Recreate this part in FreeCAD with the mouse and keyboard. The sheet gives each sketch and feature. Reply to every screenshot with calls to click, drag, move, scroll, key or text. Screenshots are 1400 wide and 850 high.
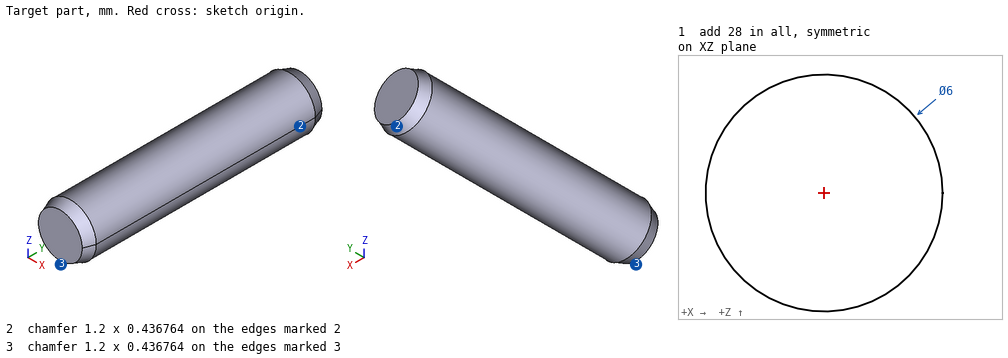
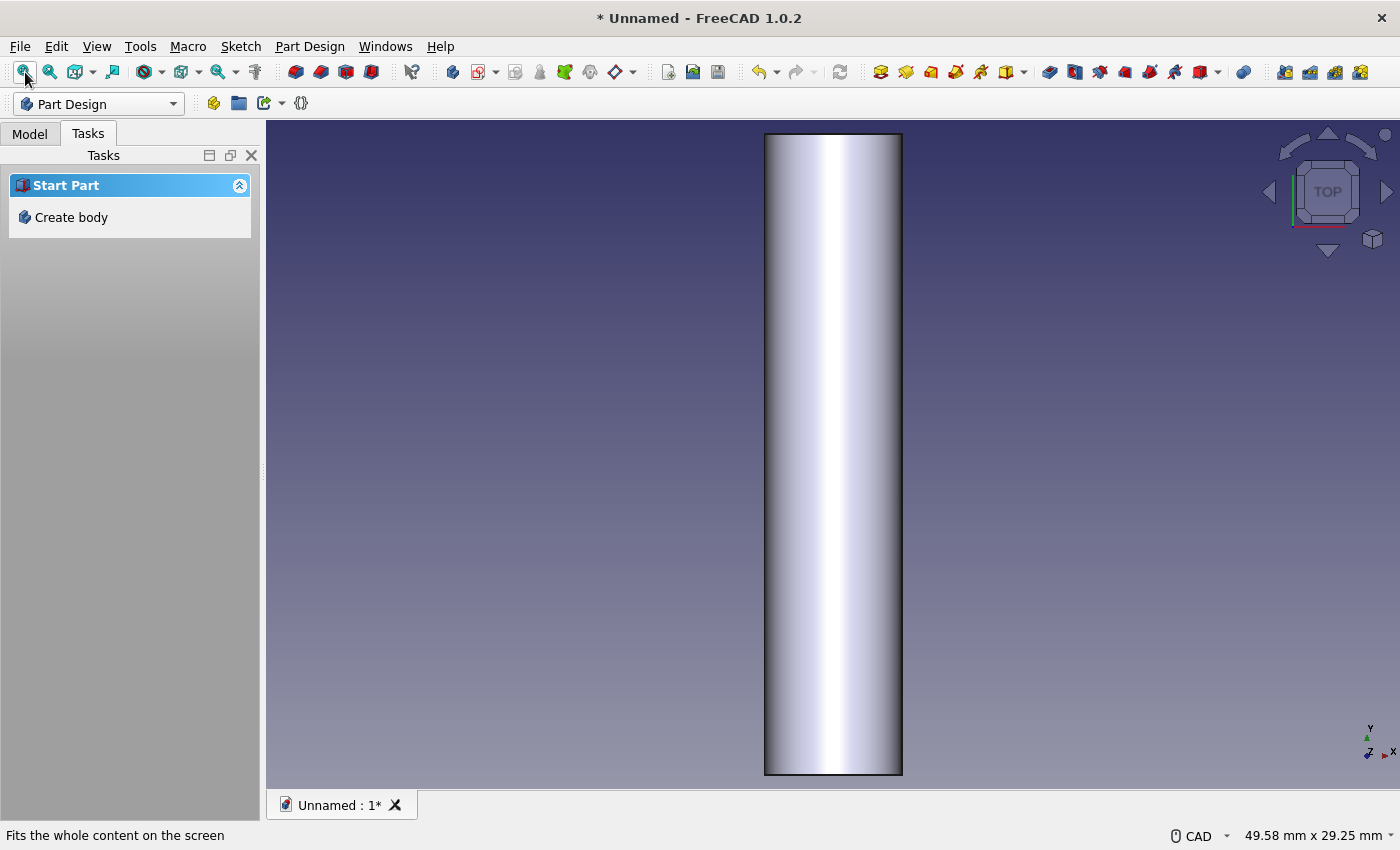
key(1)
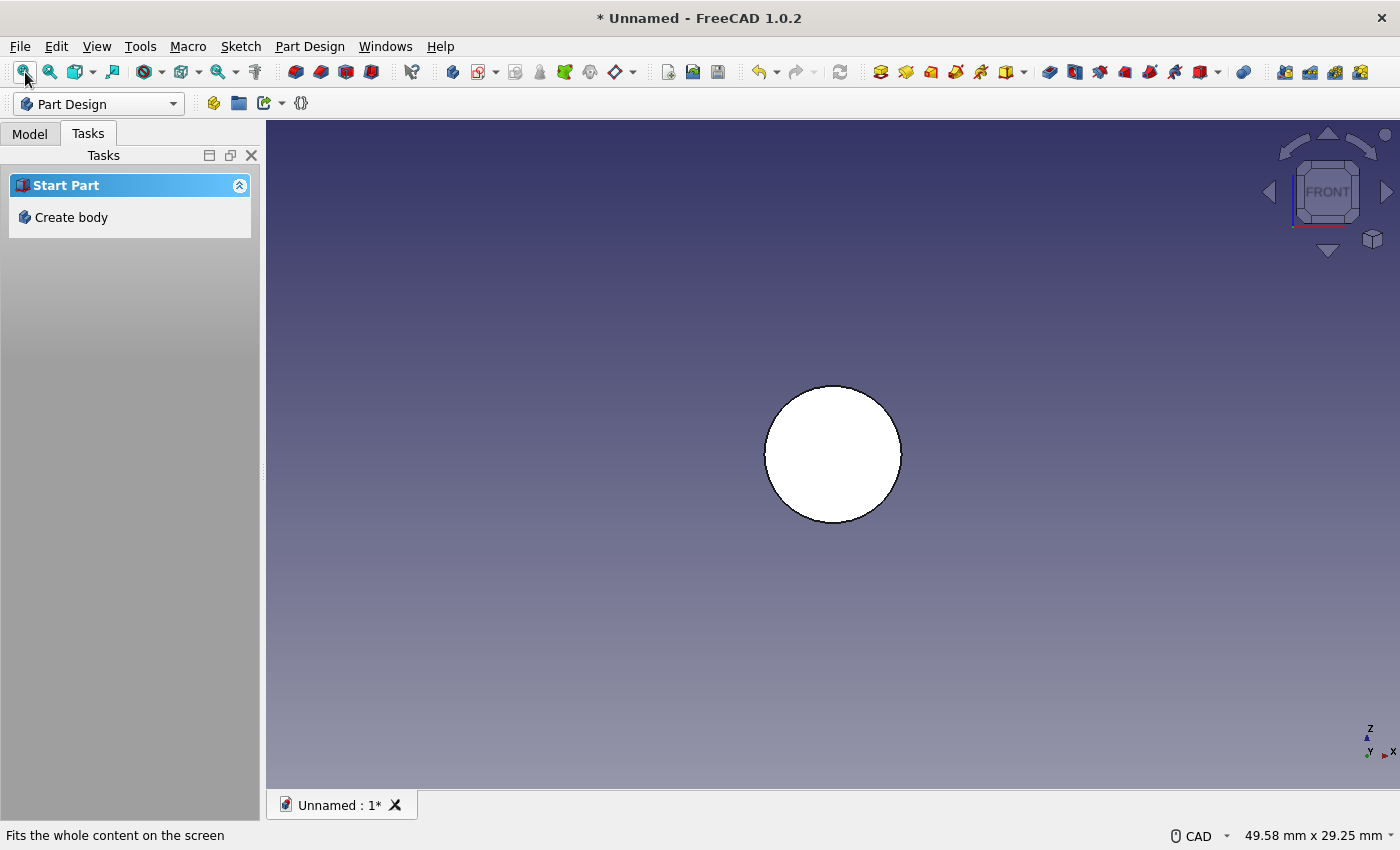
key(v)
key(f)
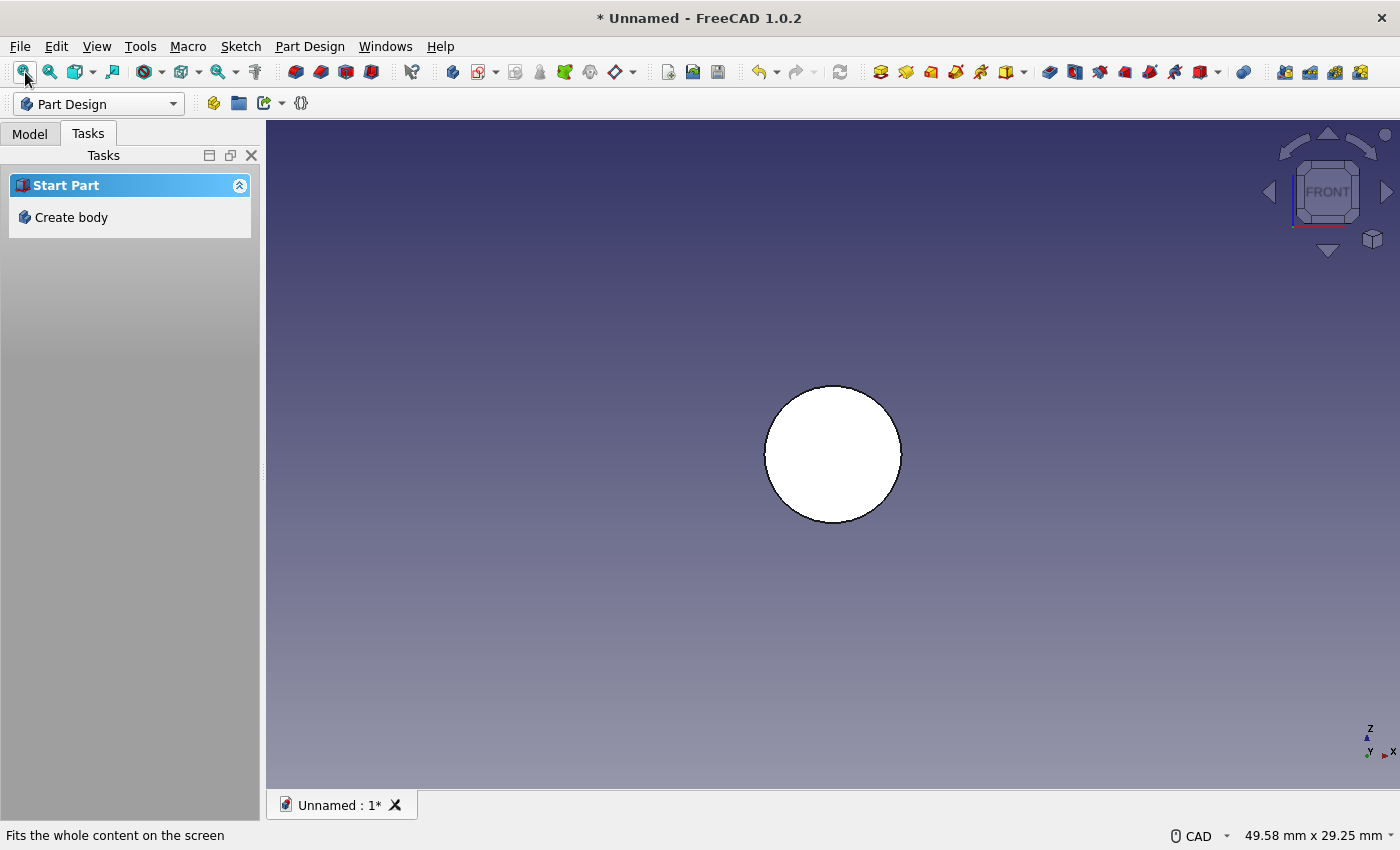
key(3)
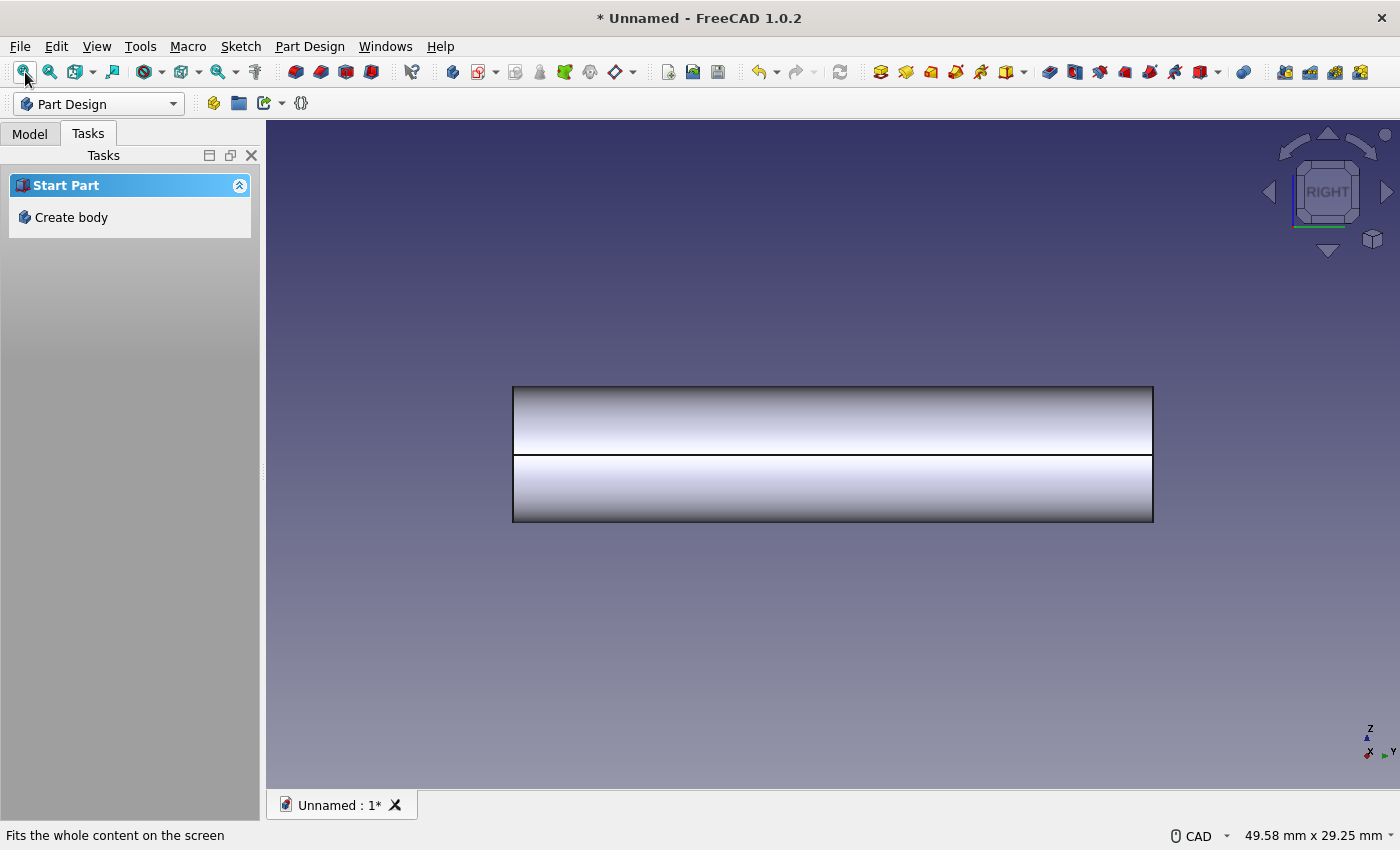
click(1153, 413)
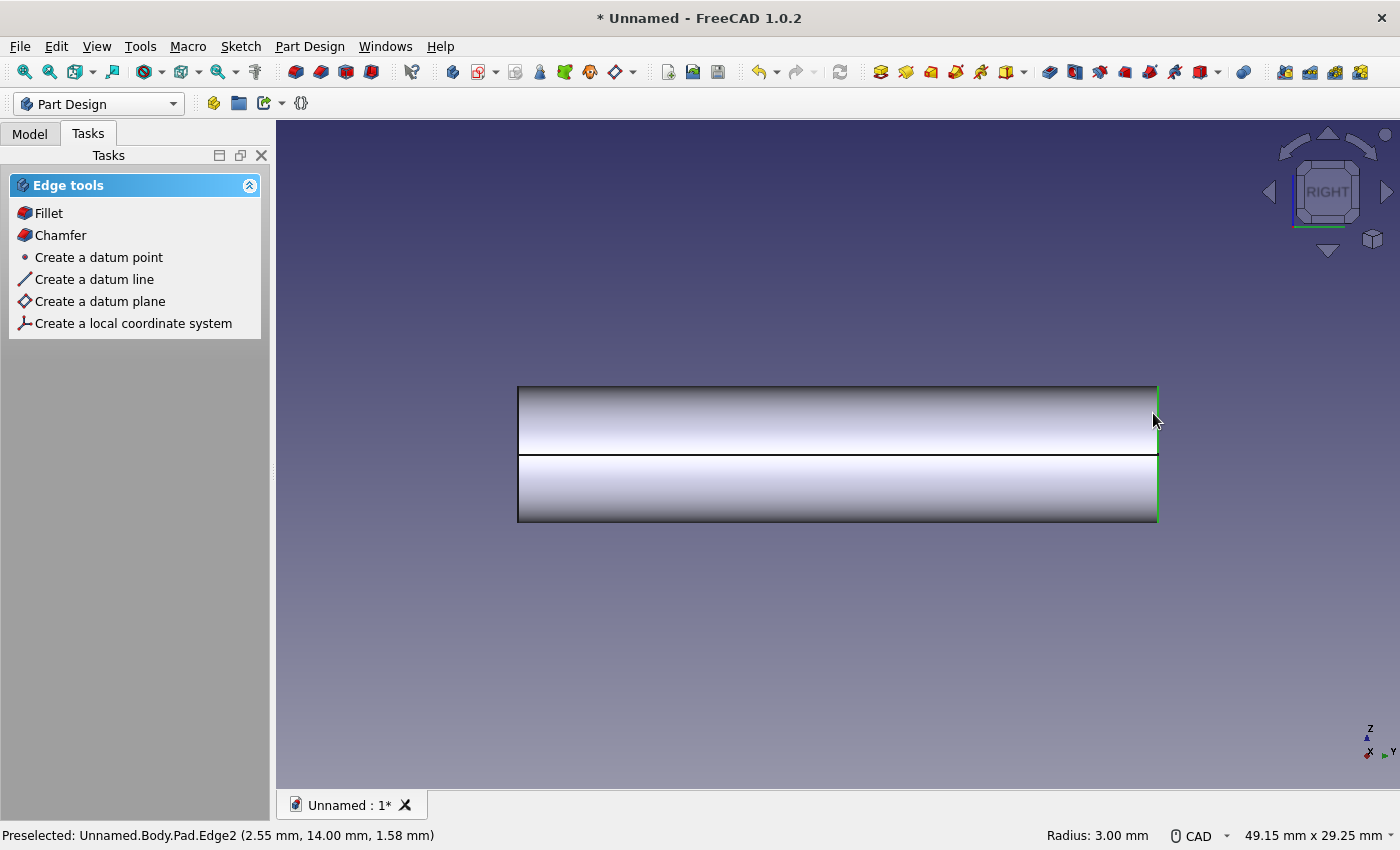
click(321, 72)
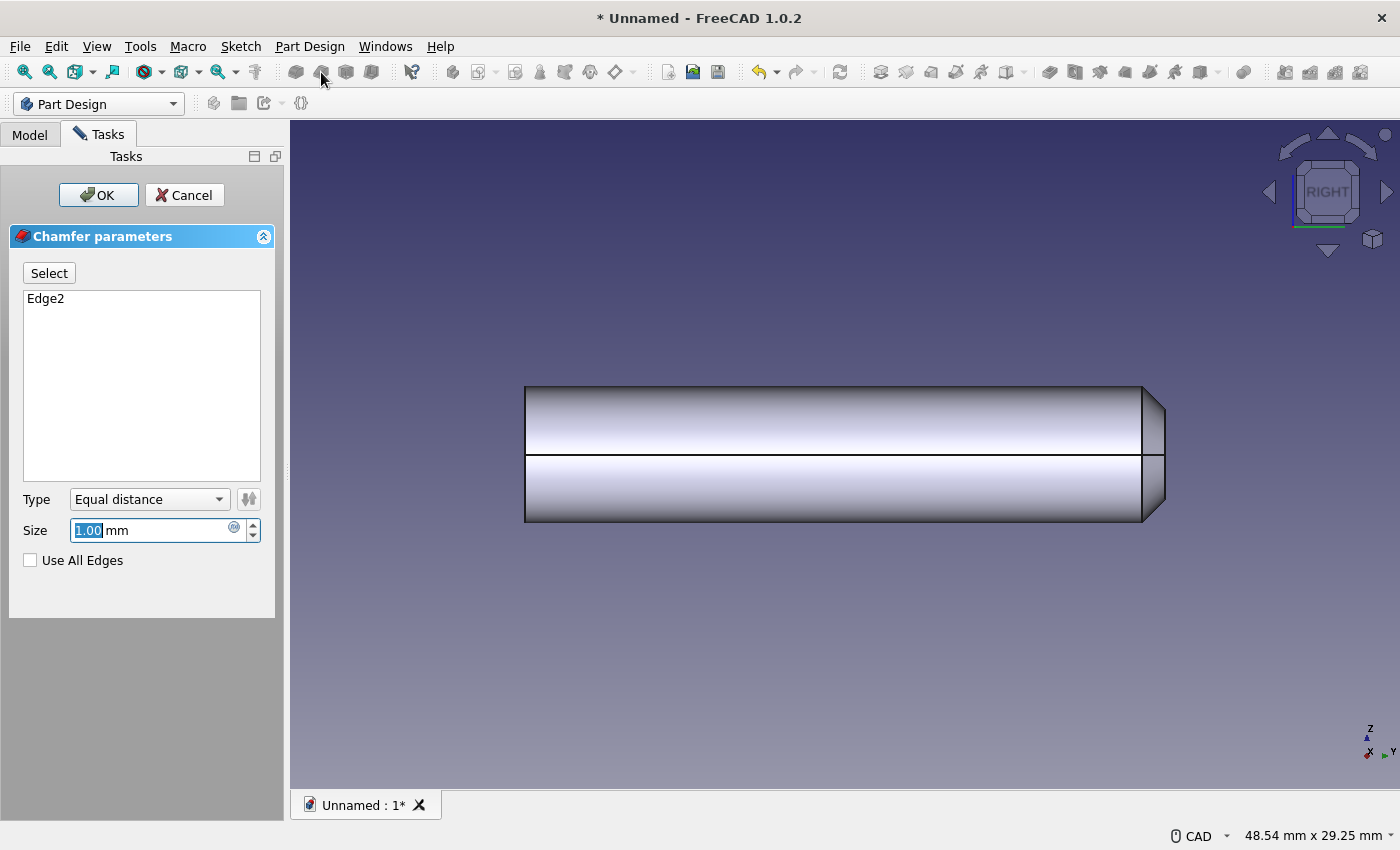
text(1.2)
key(Tab)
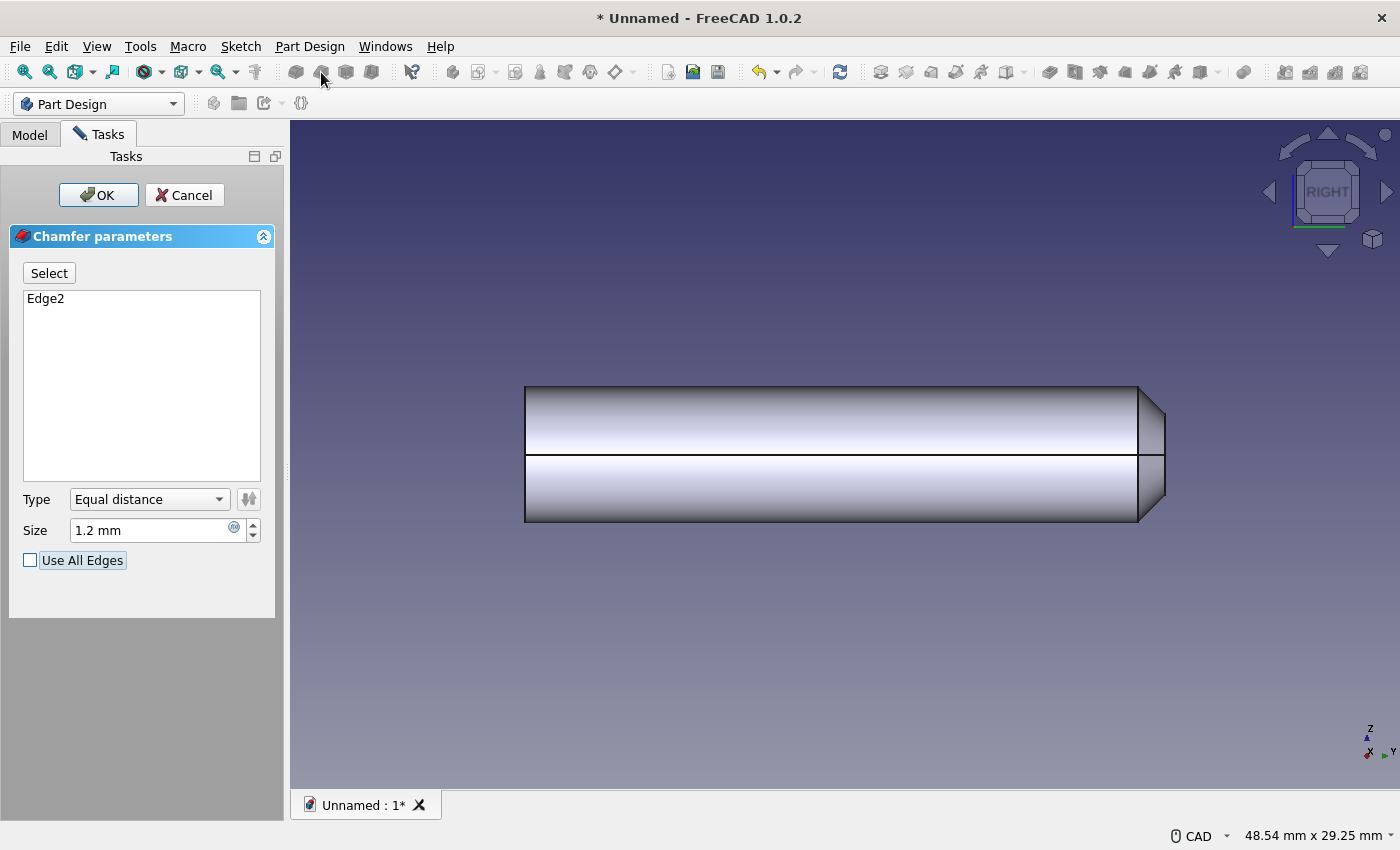
click(150, 500)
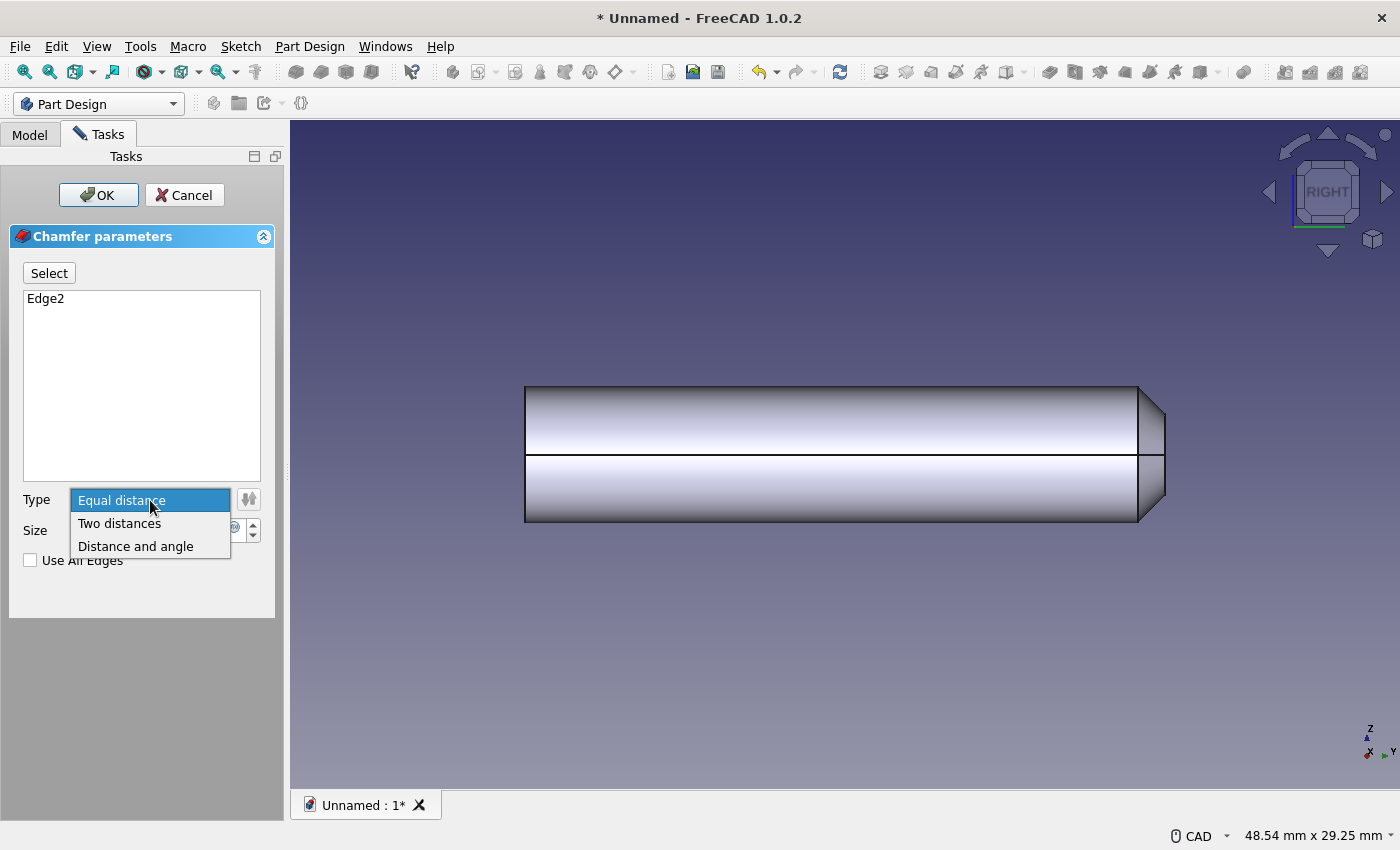
click(148, 524)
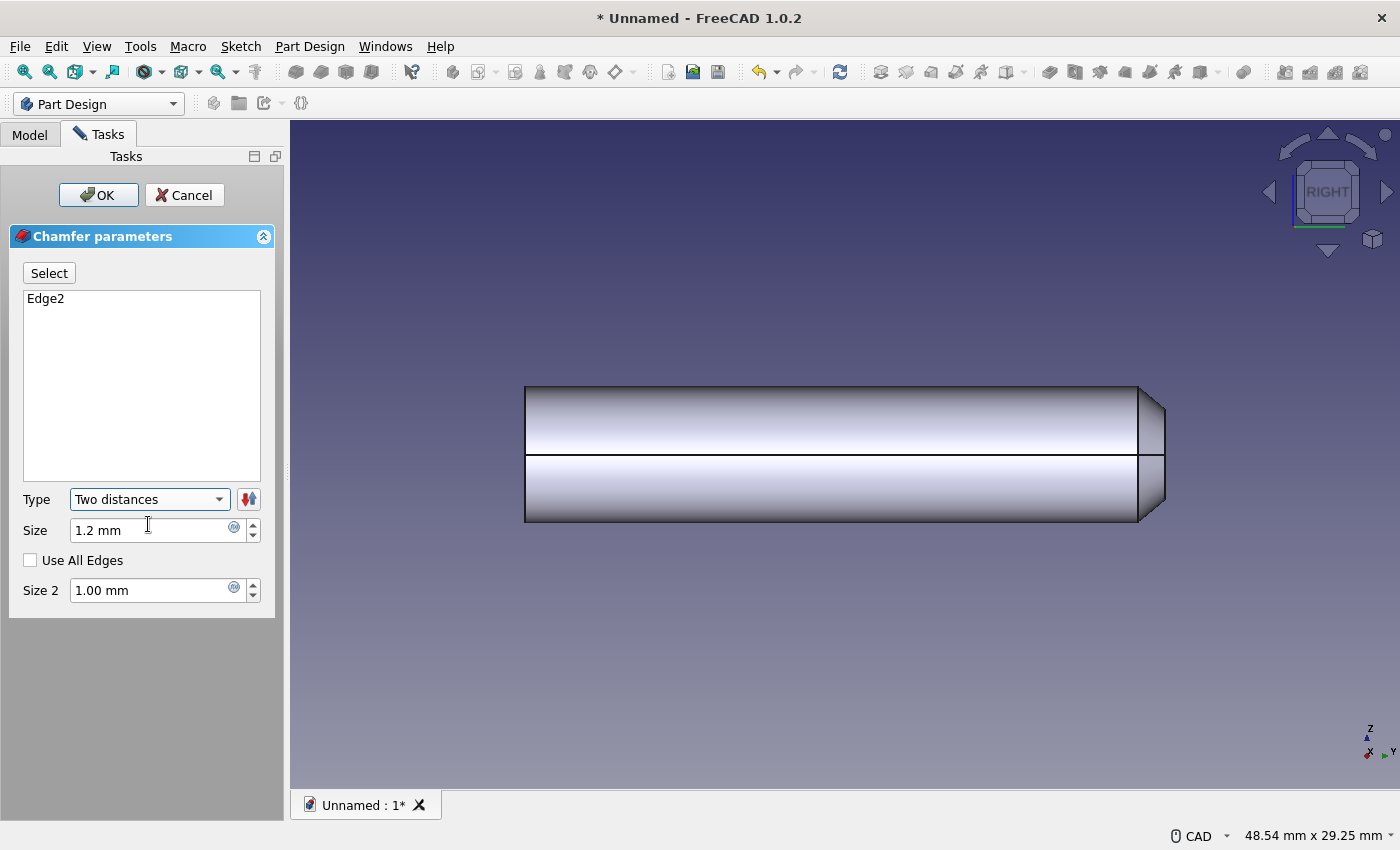
triple_click(158, 590)